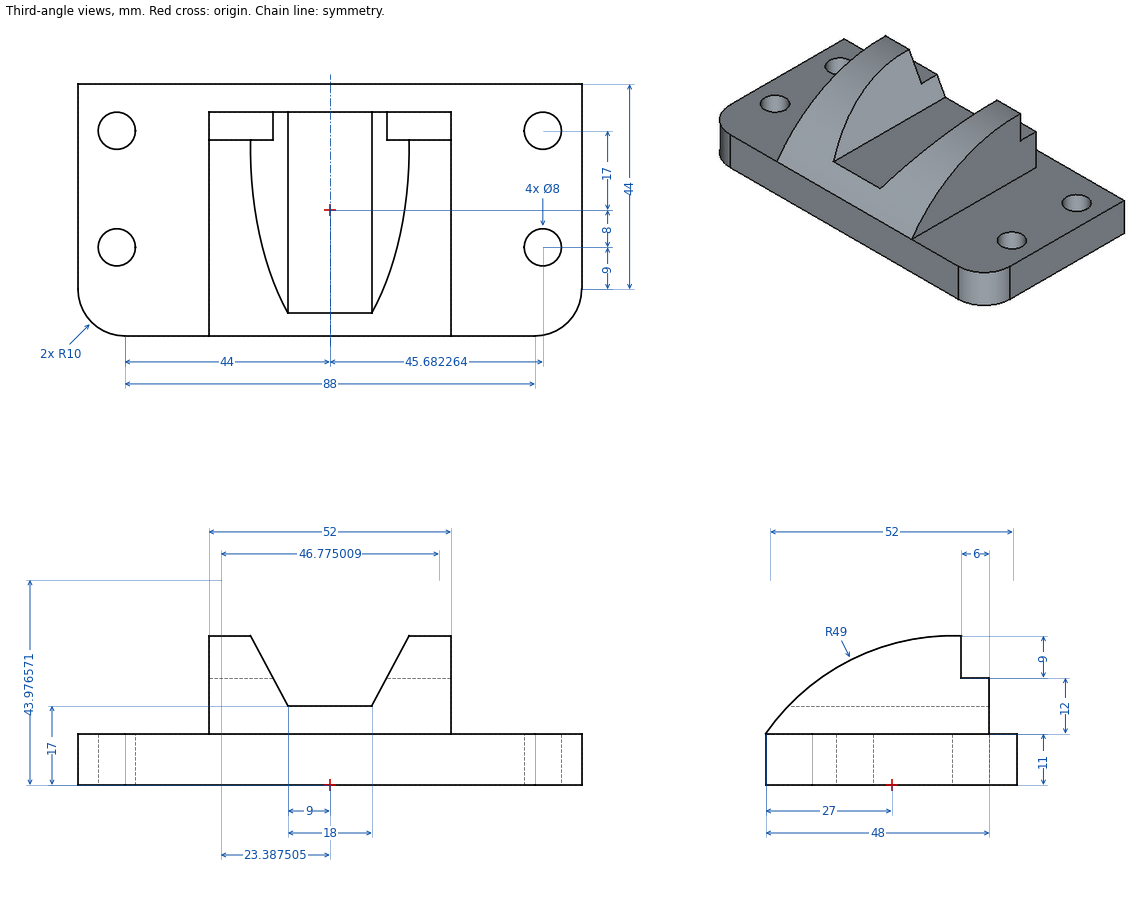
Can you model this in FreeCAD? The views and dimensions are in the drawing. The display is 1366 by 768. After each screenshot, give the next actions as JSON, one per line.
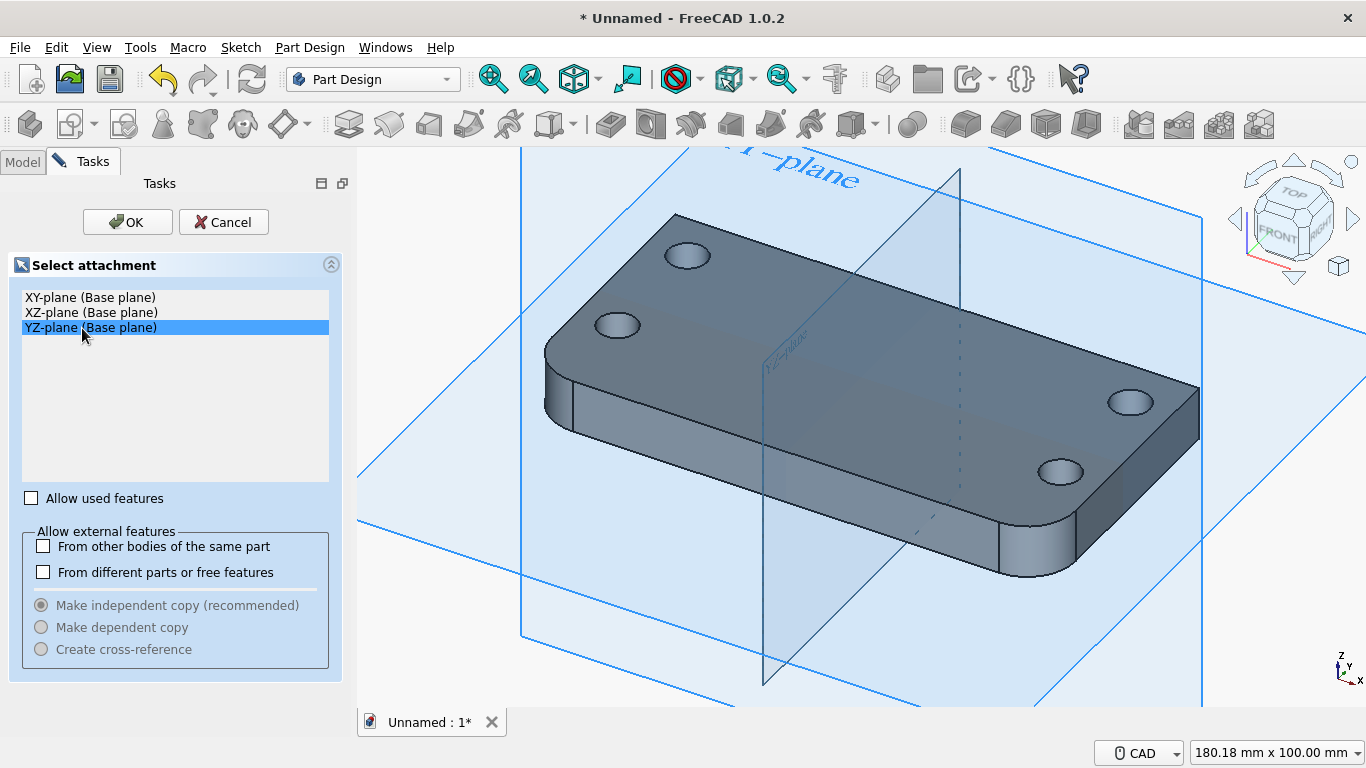
{"action": "left_click", "coordinate": [128, 222]}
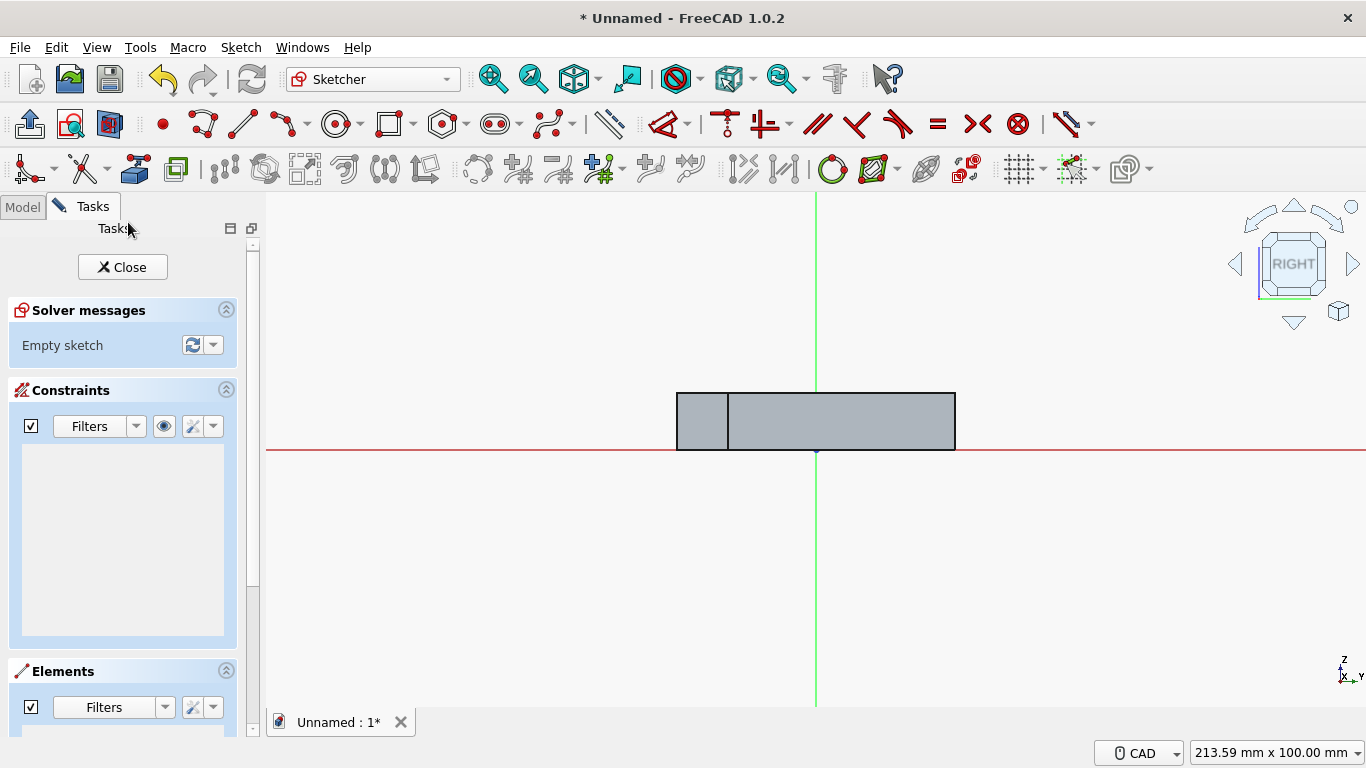
{"action": "left_click", "coordinate": [110, 124]}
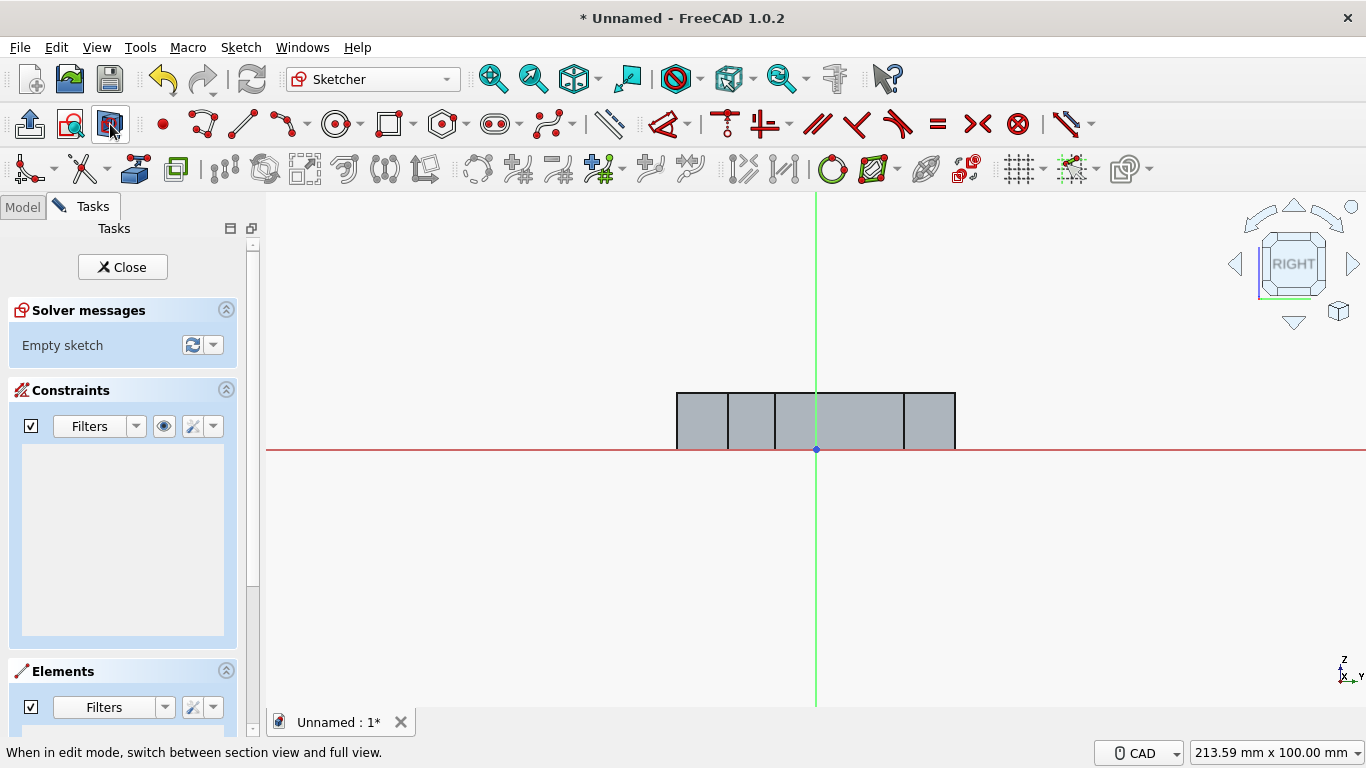
{"action": "scroll", "coordinate": [865, 267], "scroll_direction": "up", "scroll_amount": 3}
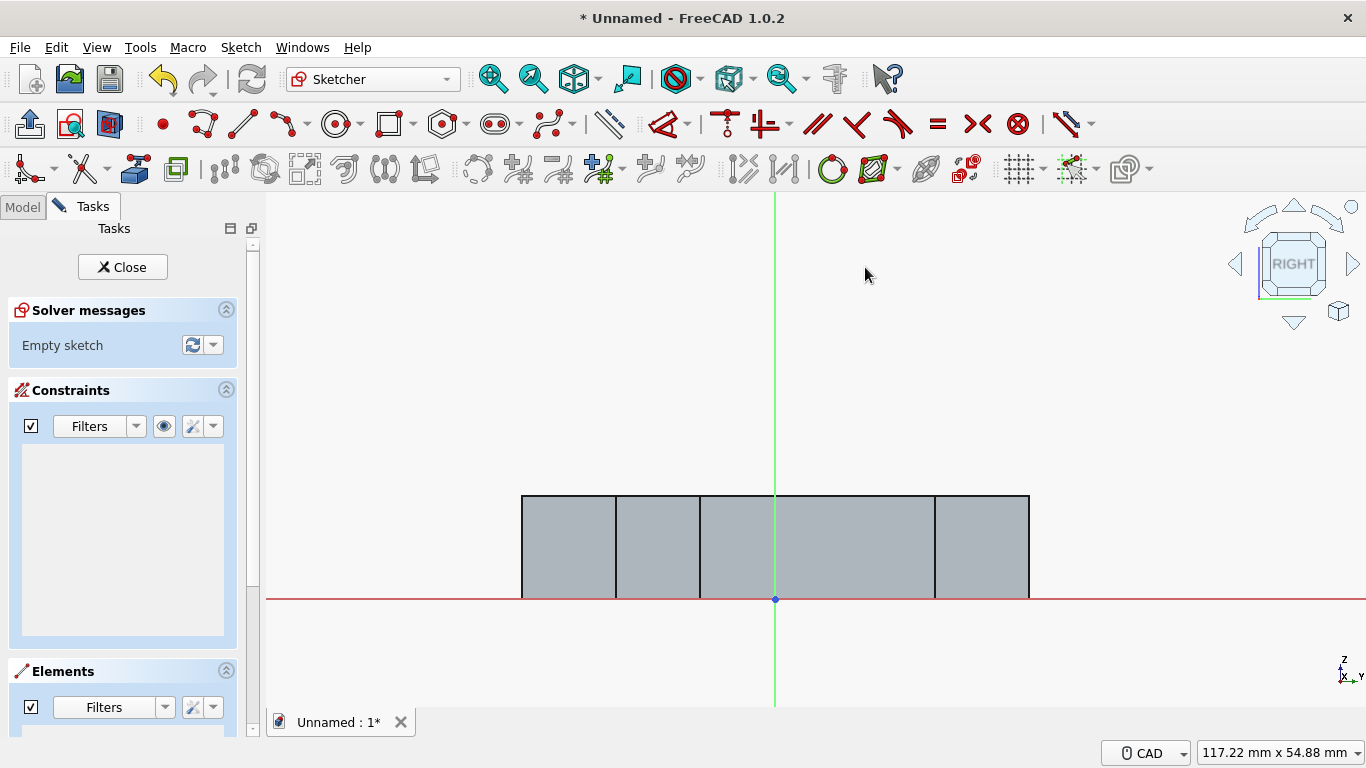
{"action": "left_click", "coordinate": [204, 124]}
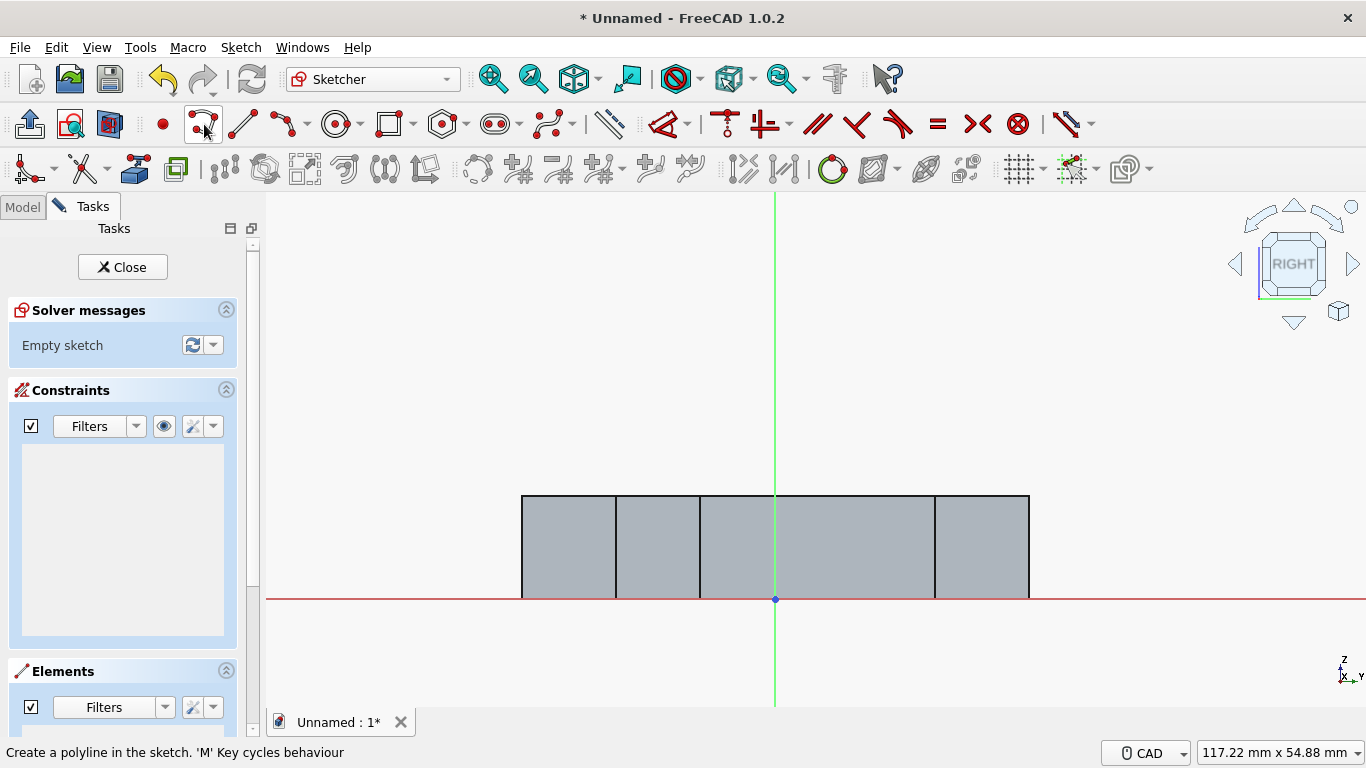
{"action": "left_click", "coordinate": [522, 496]}
{"action": "left_click", "coordinate": [972, 496]}
{"action": "left_click", "coordinate": [972, 384]}
{"action": "left_click", "coordinate": [916, 384]}
{"action": "left_click", "coordinate": [916, 299]}
{"action": "right_click", "coordinate": [916, 299]}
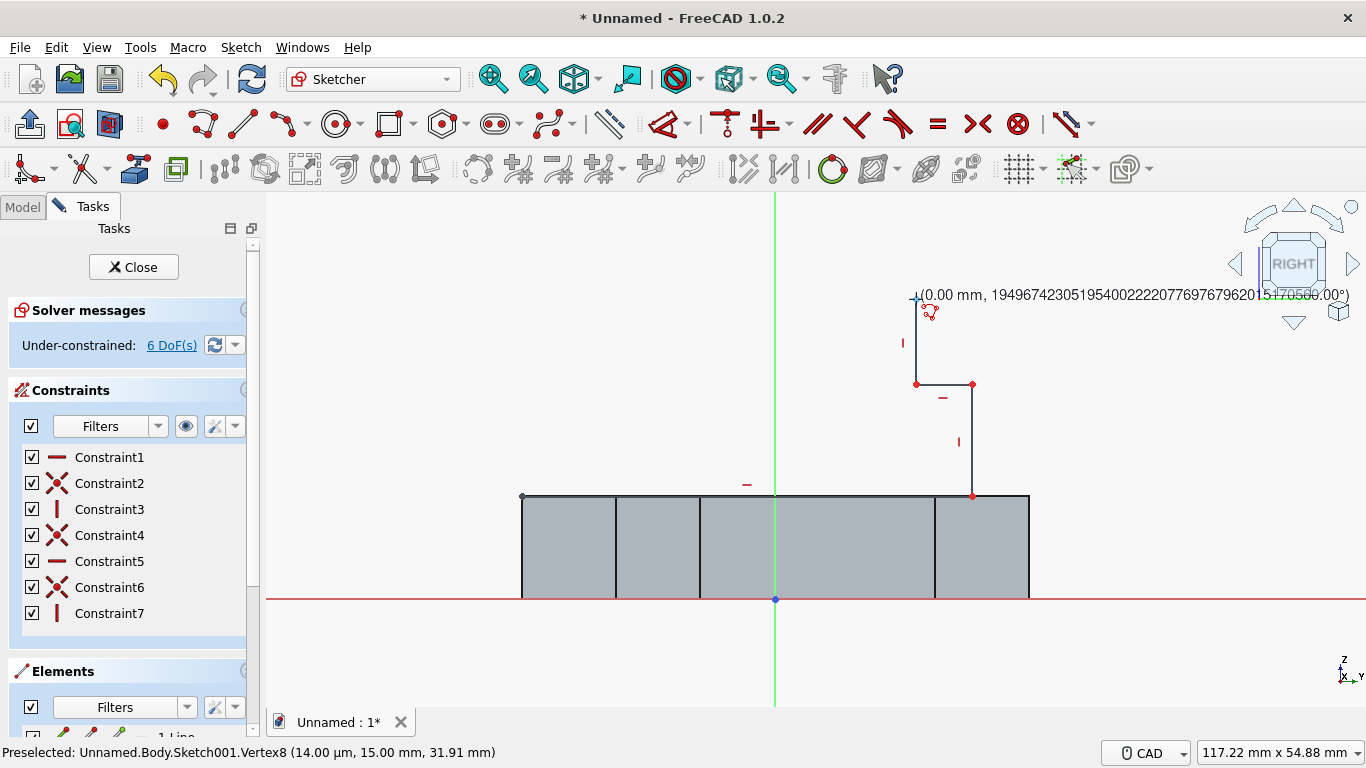
{"action": "key", "text": "g 3 a"}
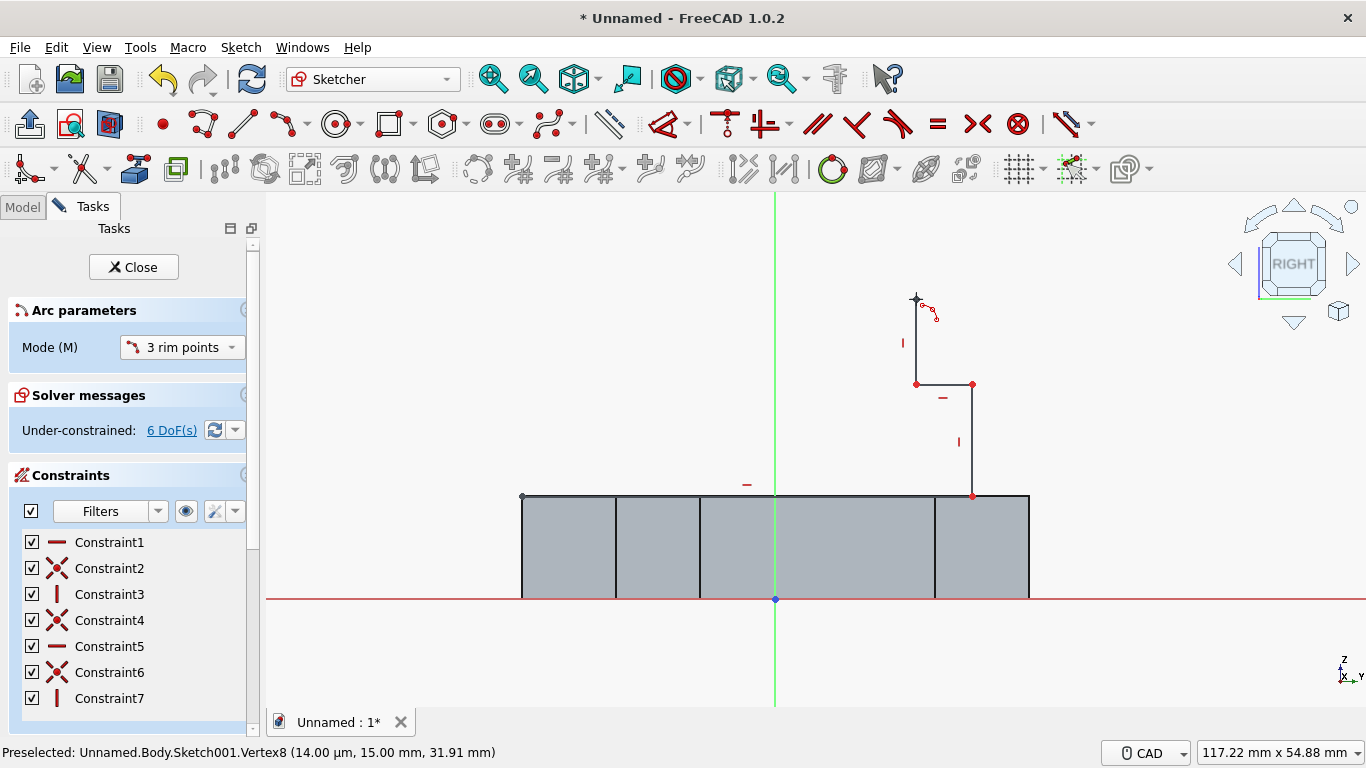
{"action": "left_click", "coordinate": [916, 300]}
{"action": "left_click", "coordinate": [522, 497]}
{"action": "left_click", "coordinate": [694, 347]}
{"action": "key", "text": "Escape"}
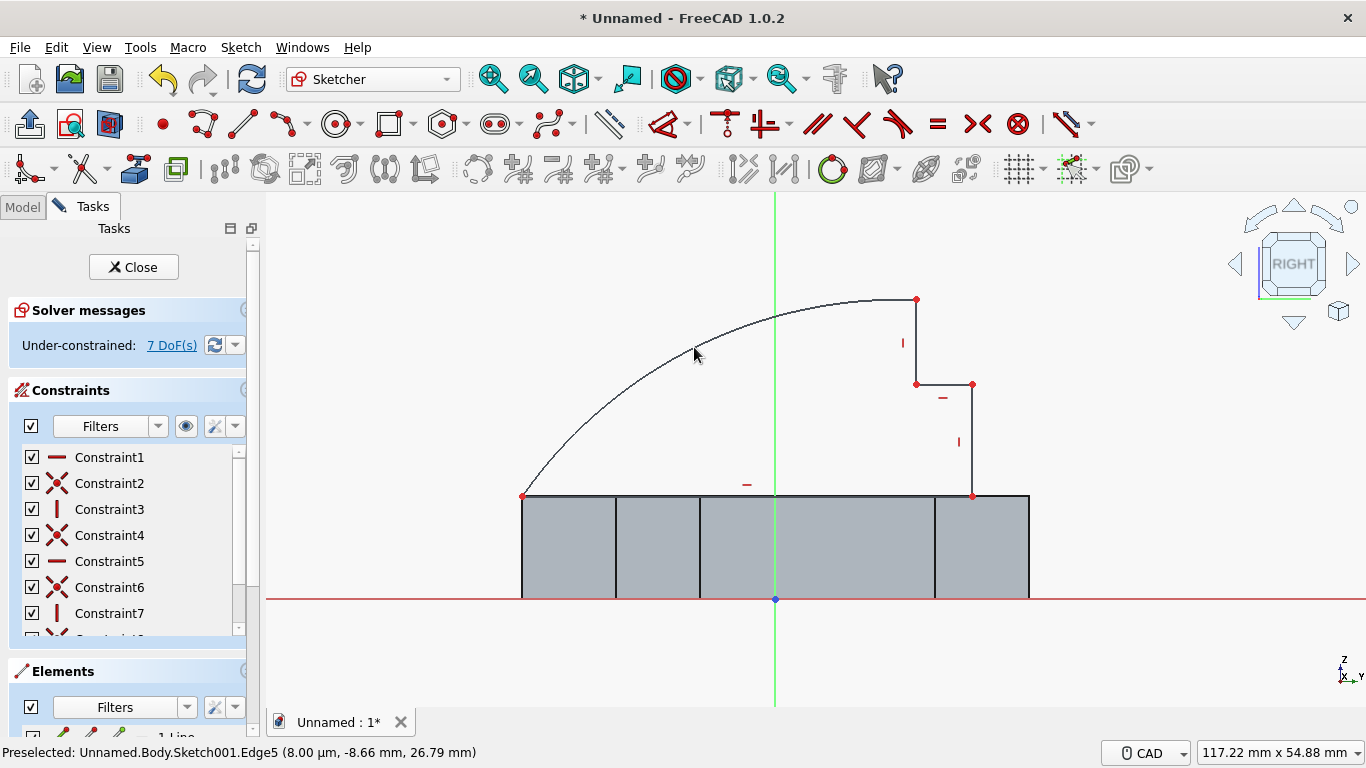
{"action": "left_click", "coordinate": [664, 124]}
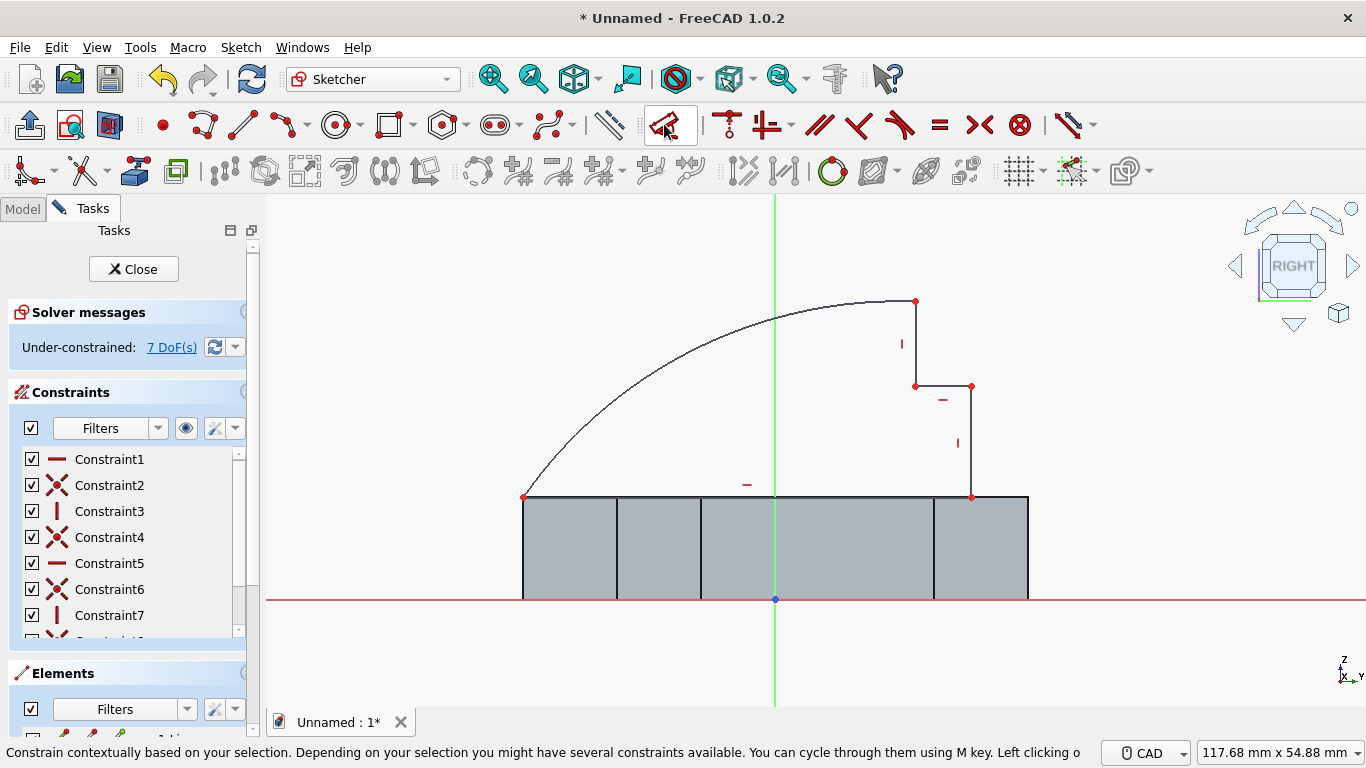
{"action": "left_click", "coordinate": [617, 398]}
{"action": "left_click", "coordinate": [597, 373]}